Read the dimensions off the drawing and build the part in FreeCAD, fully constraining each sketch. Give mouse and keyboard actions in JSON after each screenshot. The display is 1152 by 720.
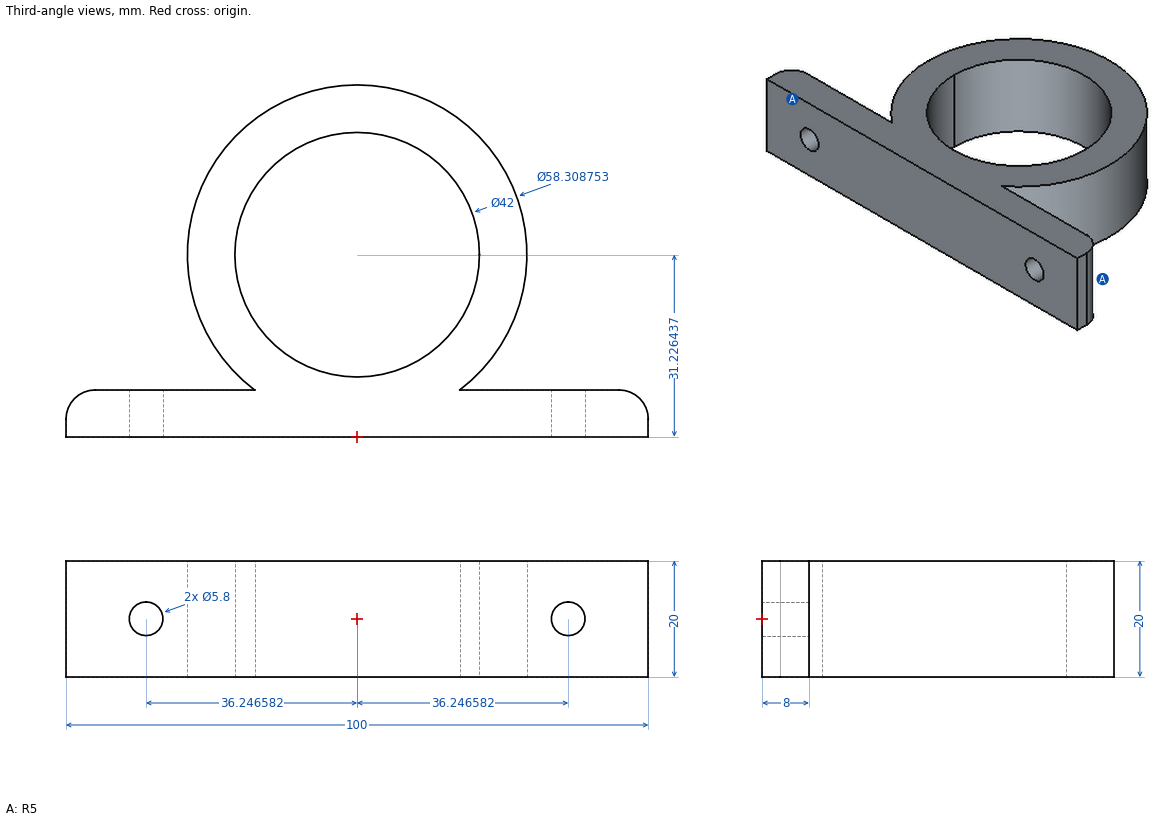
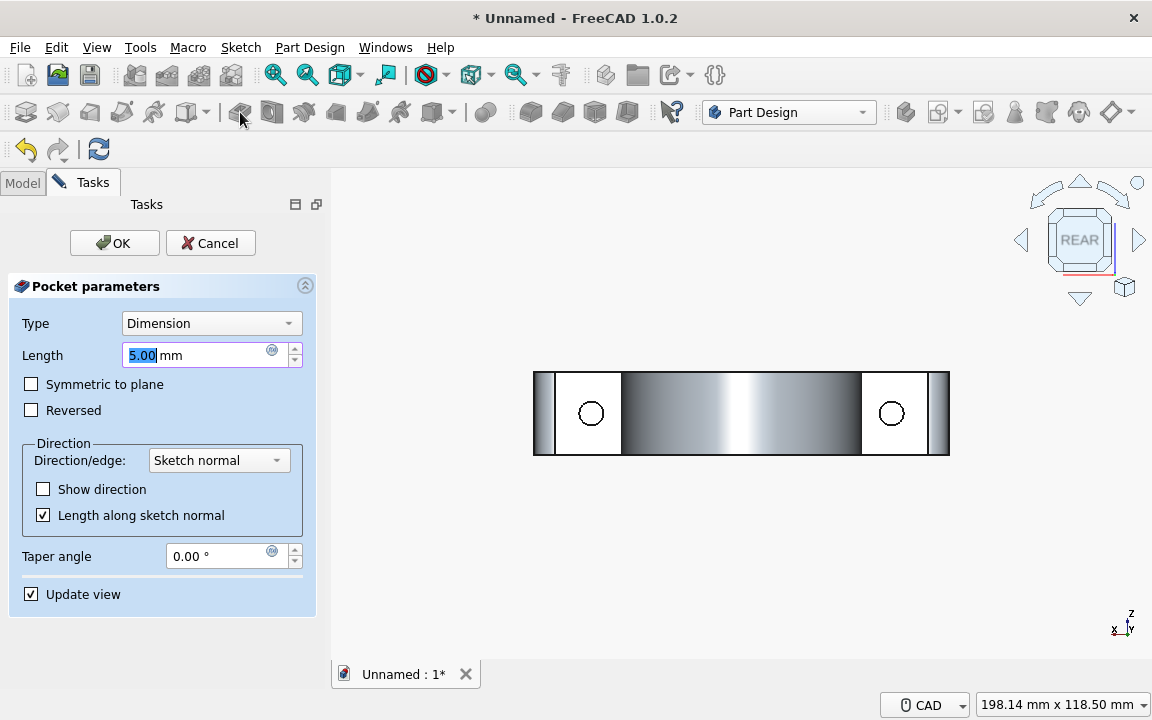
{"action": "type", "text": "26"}
{"action": "key", "text": "Tab"}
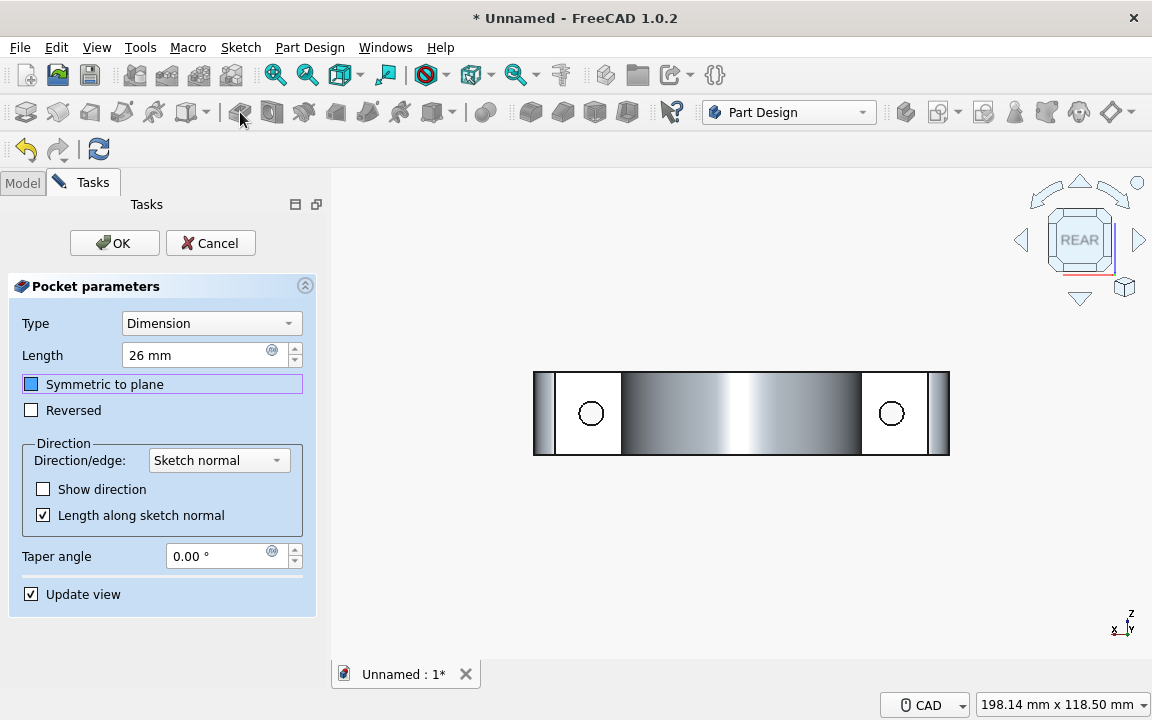
{"action": "left_click", "coordinate": [115, 243]}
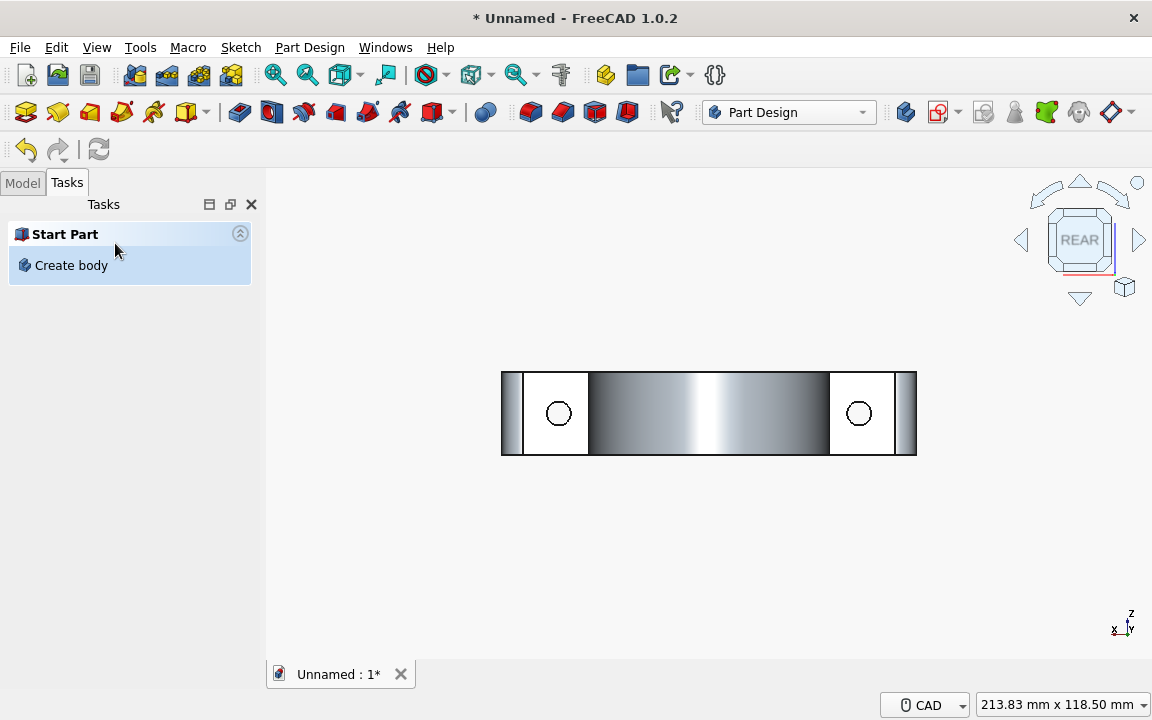
{"action": "key", "text": "0"}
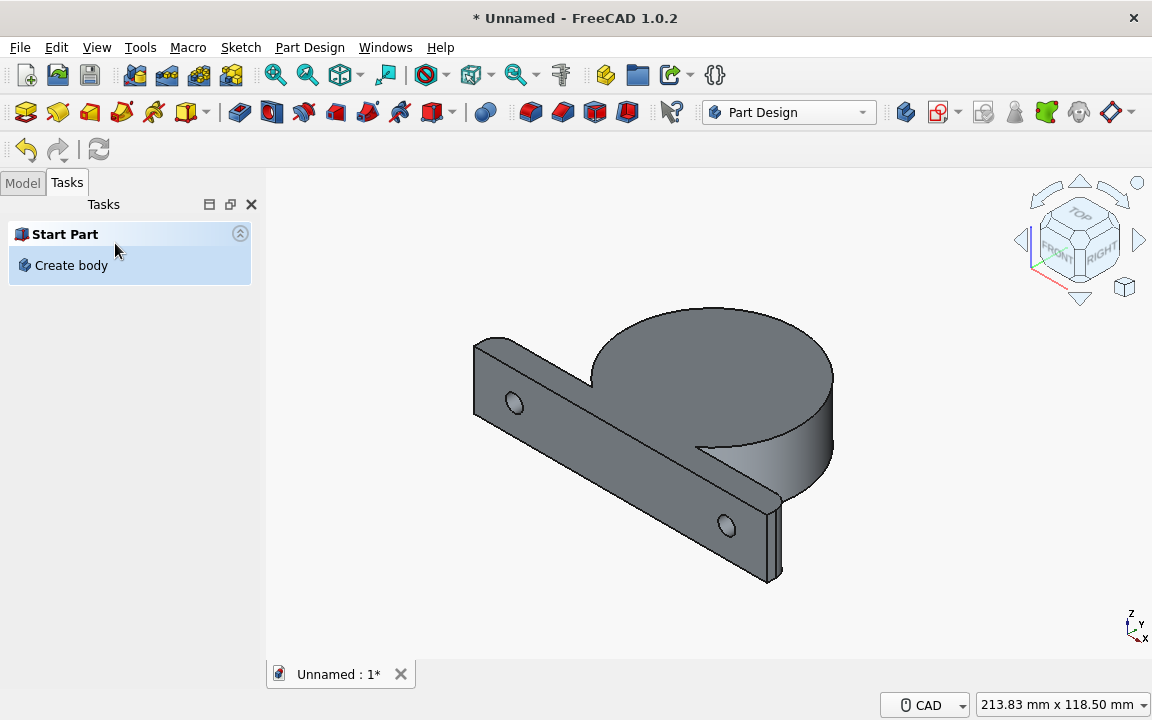
{"action": "left_click", "coordinate": [709, 379]}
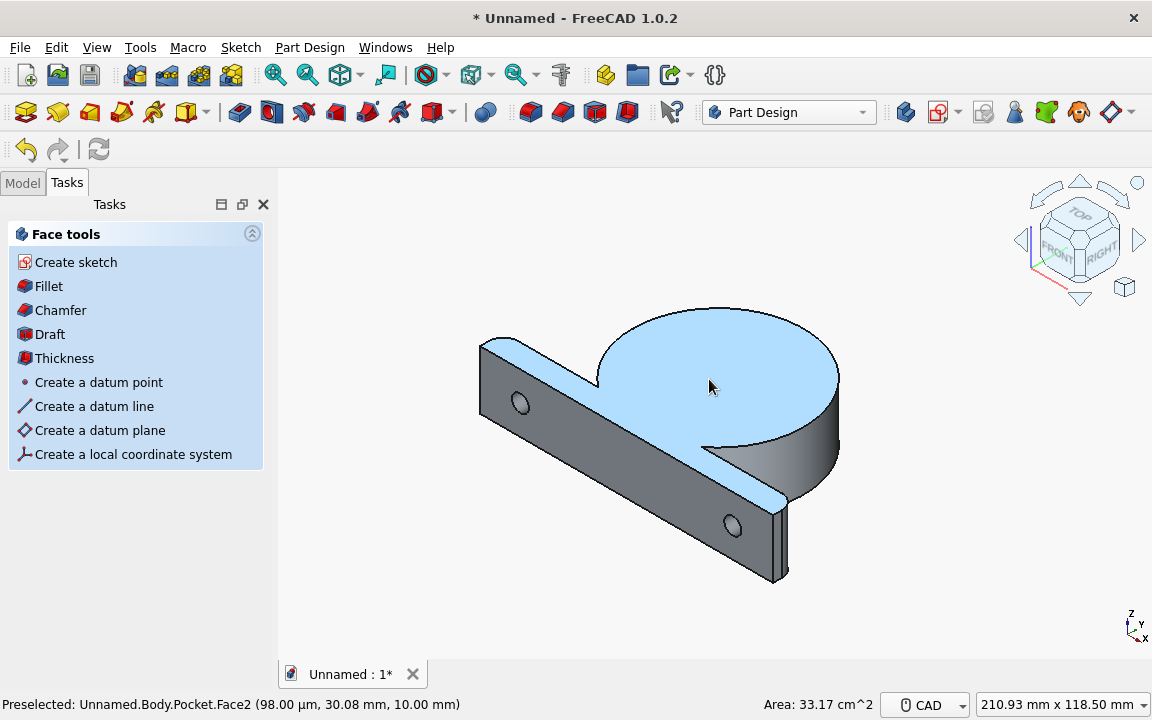
{"action": "left_click", "coordinate": [938, 112]}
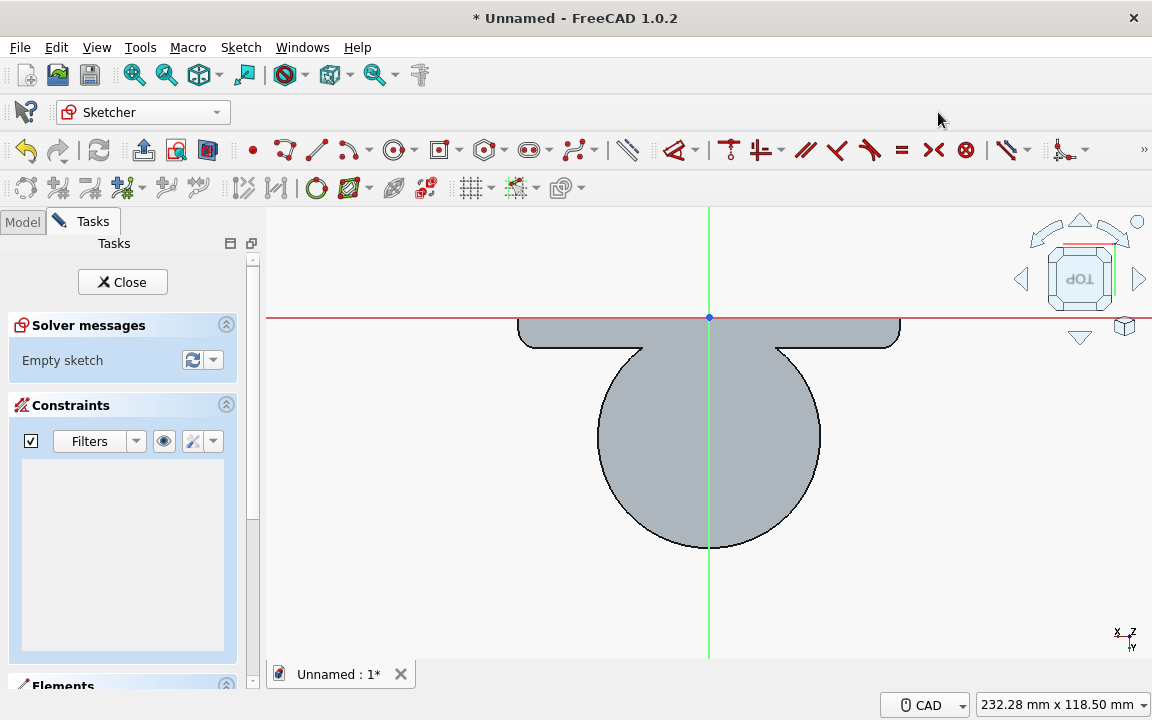
{"action": "scroll", "coordinate": [848, 386], "scroll_direction": "up", "scroll_amount": 2}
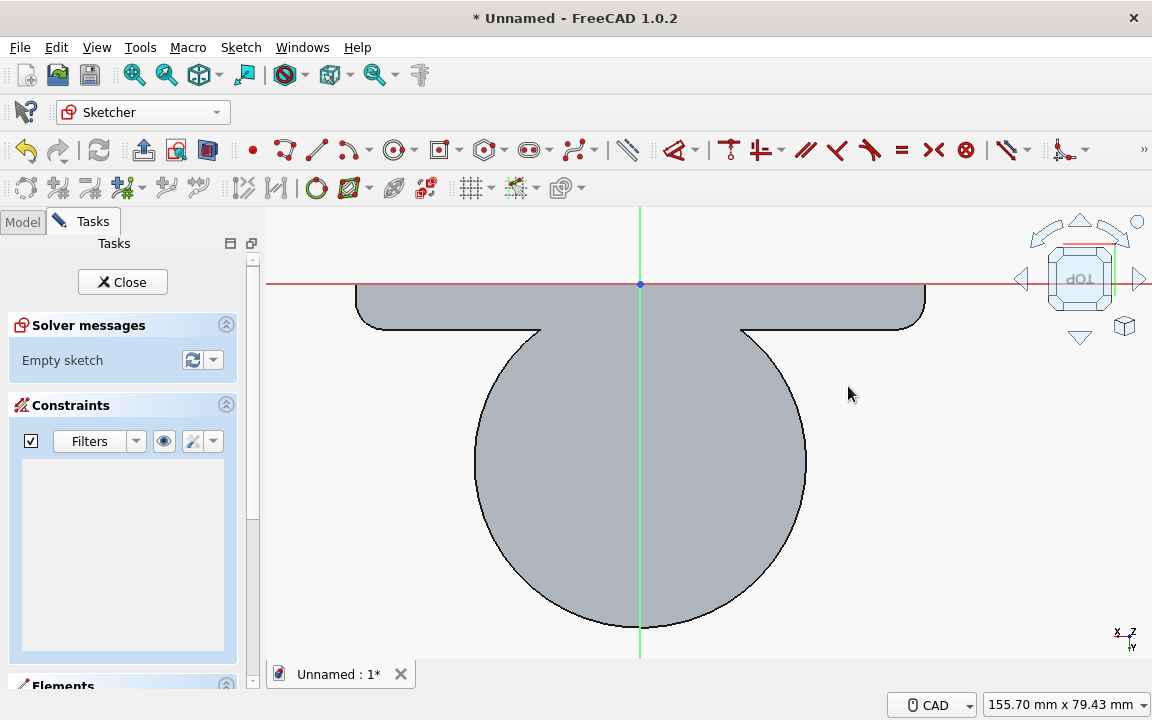
{"action": "left_click", "coordinate": [394, 150]}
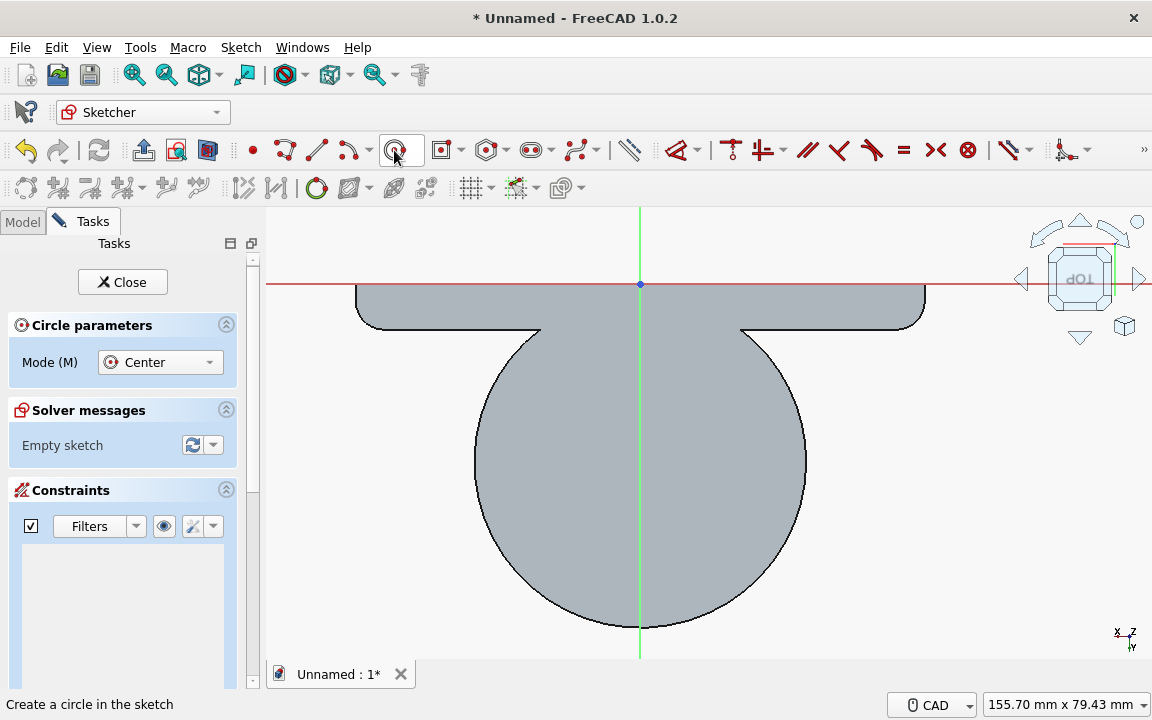
{"action": "left_click", "coordinate": [640, 462]}
{"action": "left_click", "coordinate": [725, 377]}
{"action": "key", "text": "Escape"}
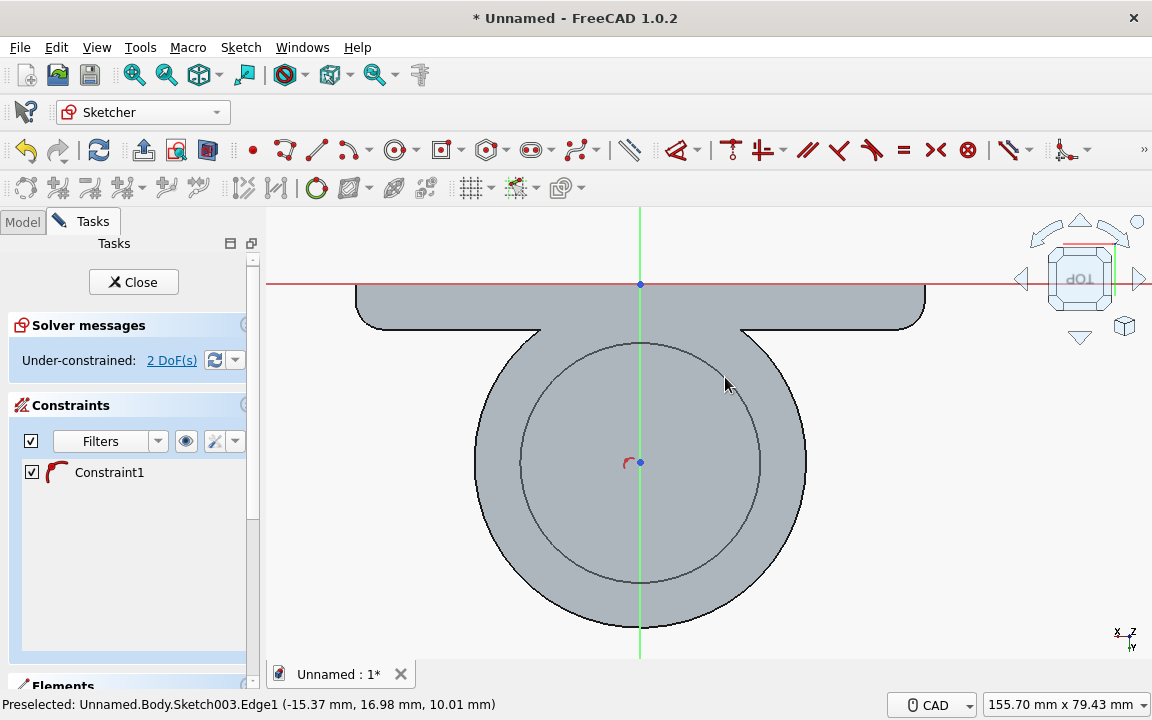
{"action": "left_click", "coordinate": [676, 150]}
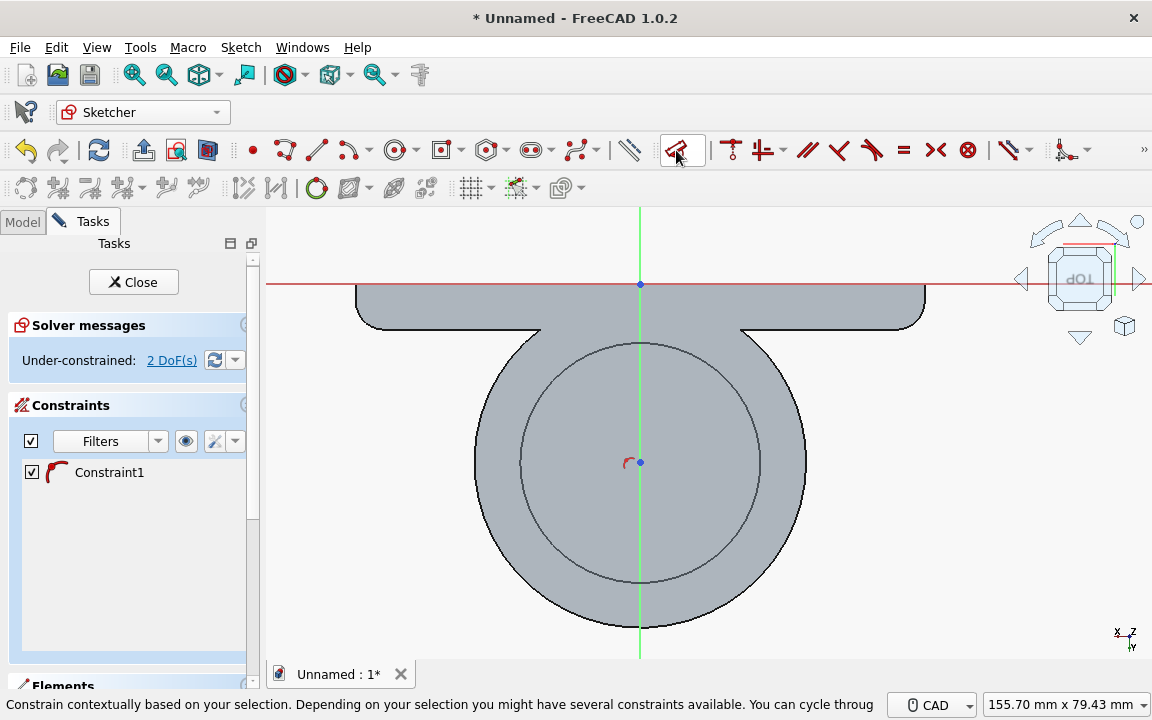
{"action": "left_click", "coordinate": [725, 378]}
{"action": "left_click", "coordinate": [748, 355]}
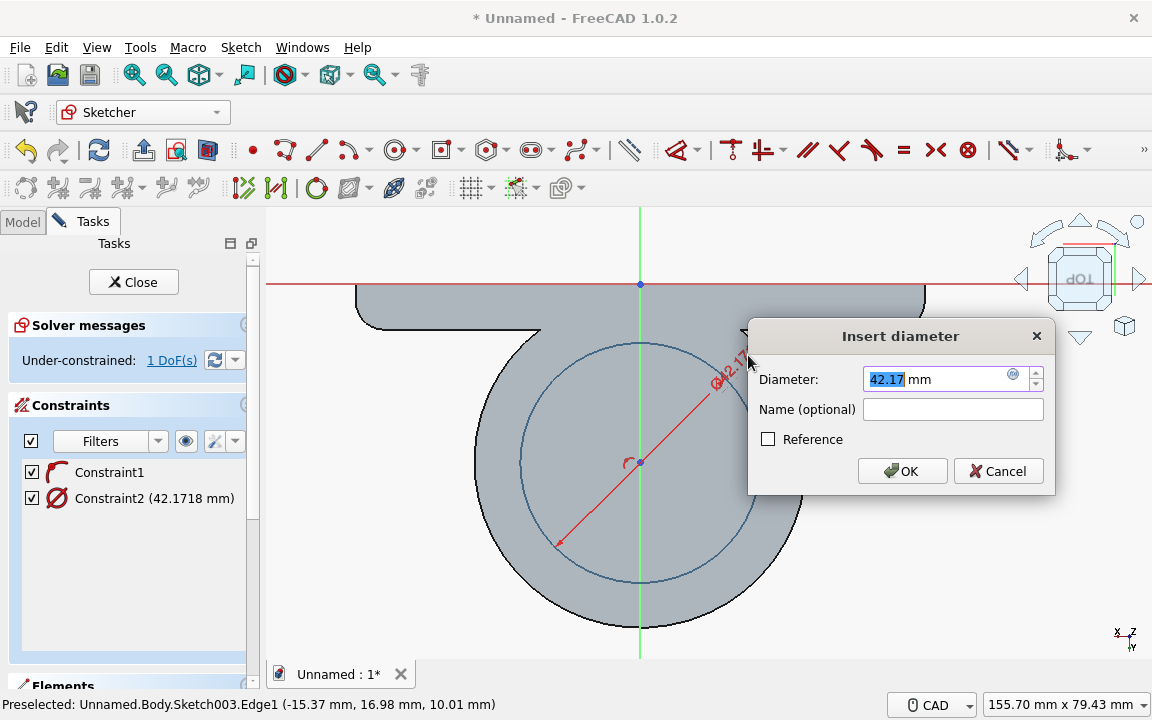
{"action": "type", "text": "42"}
{"action": "key", "text": "Return"}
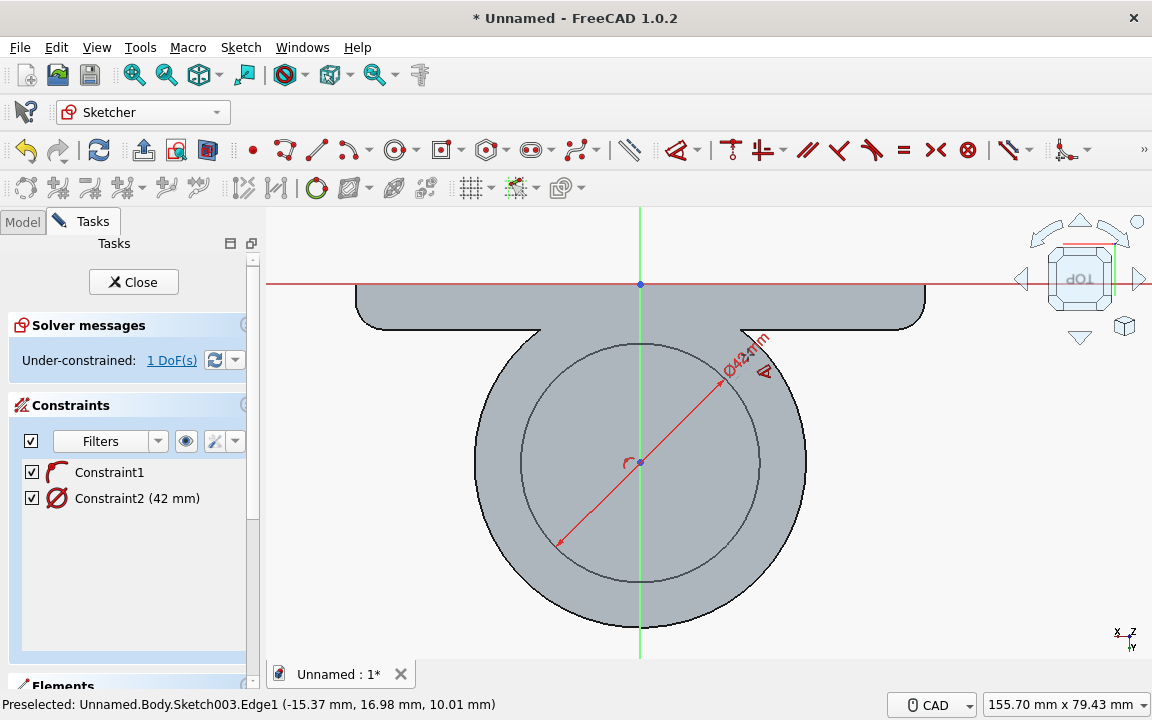
{"action": "left_click", "coordinate": [640, 463]}
{"action": "left_click", "coordinate": [674, 374]}